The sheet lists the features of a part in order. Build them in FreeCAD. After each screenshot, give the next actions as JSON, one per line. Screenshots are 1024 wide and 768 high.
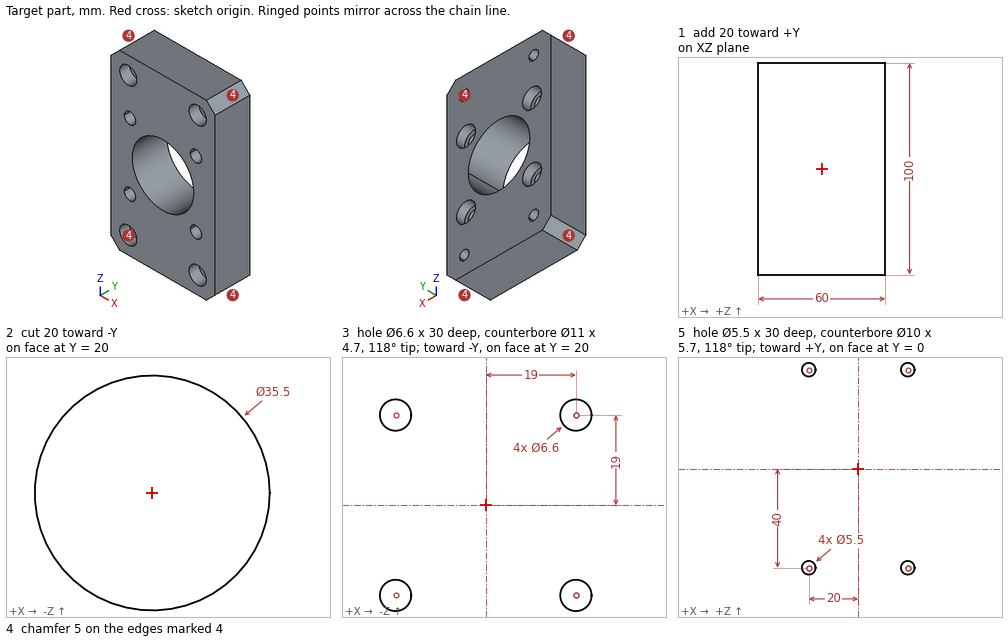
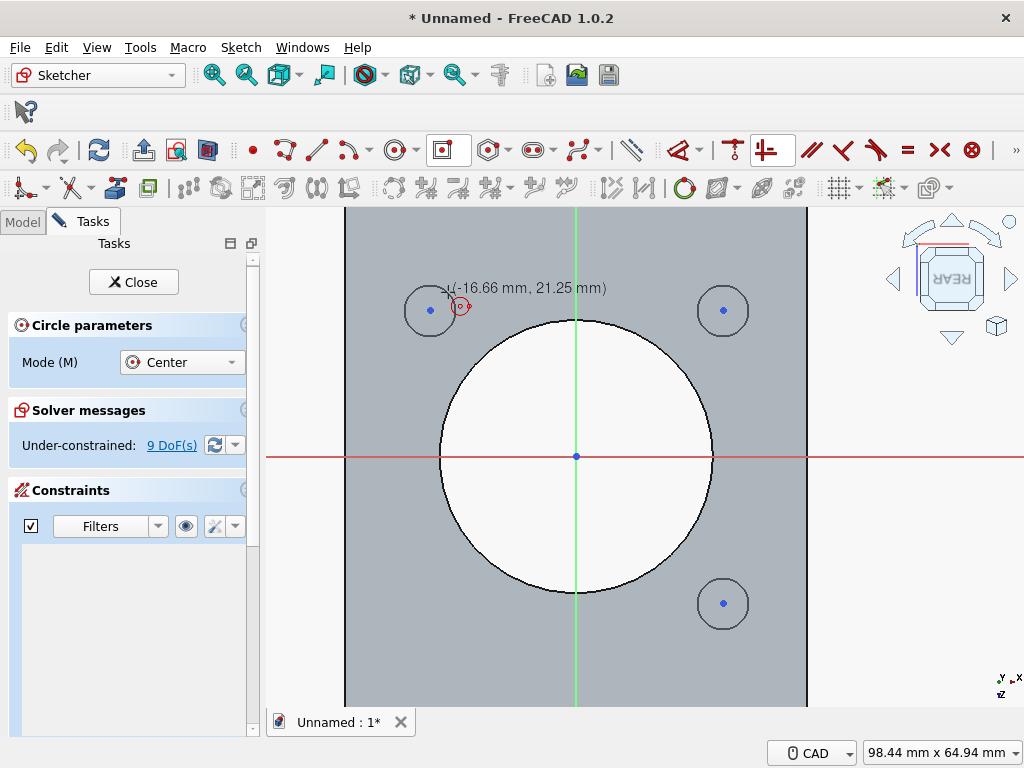
{"action": "left_click", "coordinate": [430, 603]}
{"action": "left_click", "coordinate": [448, 585]}
{"action": "key", "text": "Escape"}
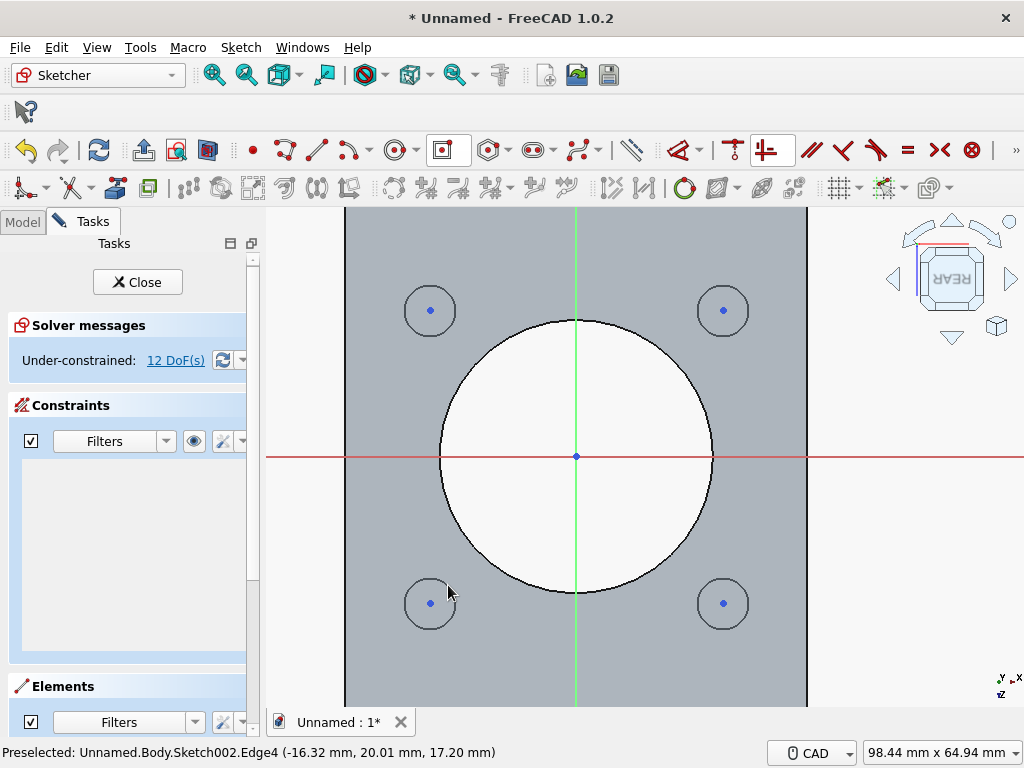
{"action": "left_click", "coordinate": [741, 293]}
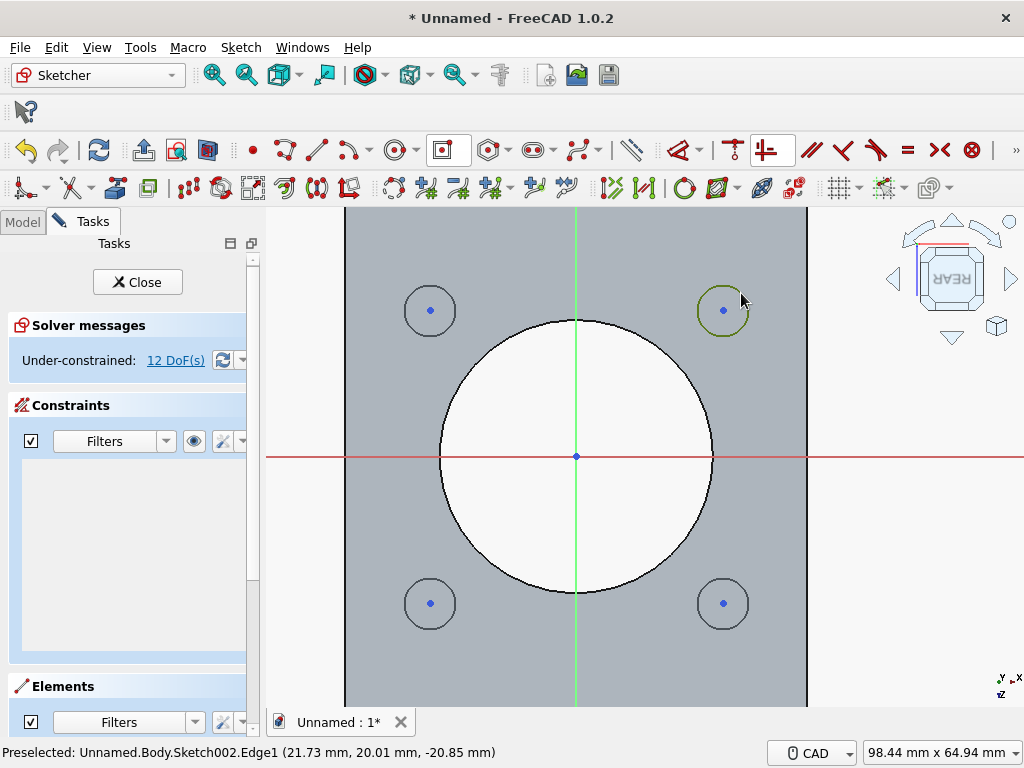
{"action": "left_click", "coordinate": [741, 586]}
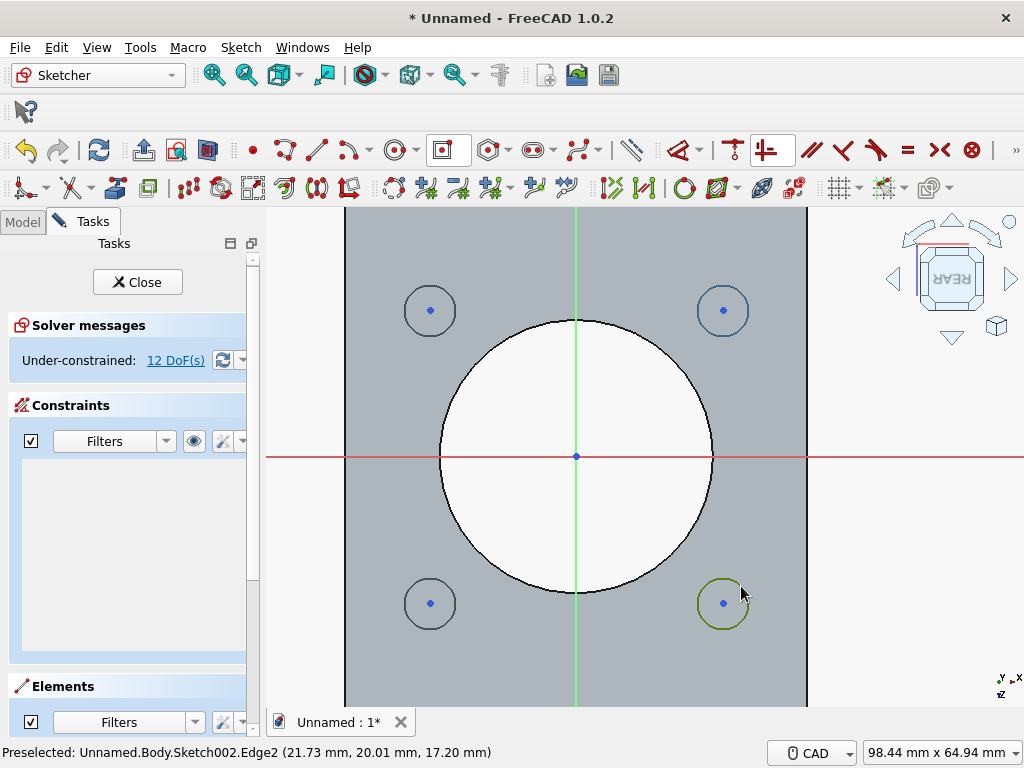
{"action": "left_click", "coordinate": [448, 293]}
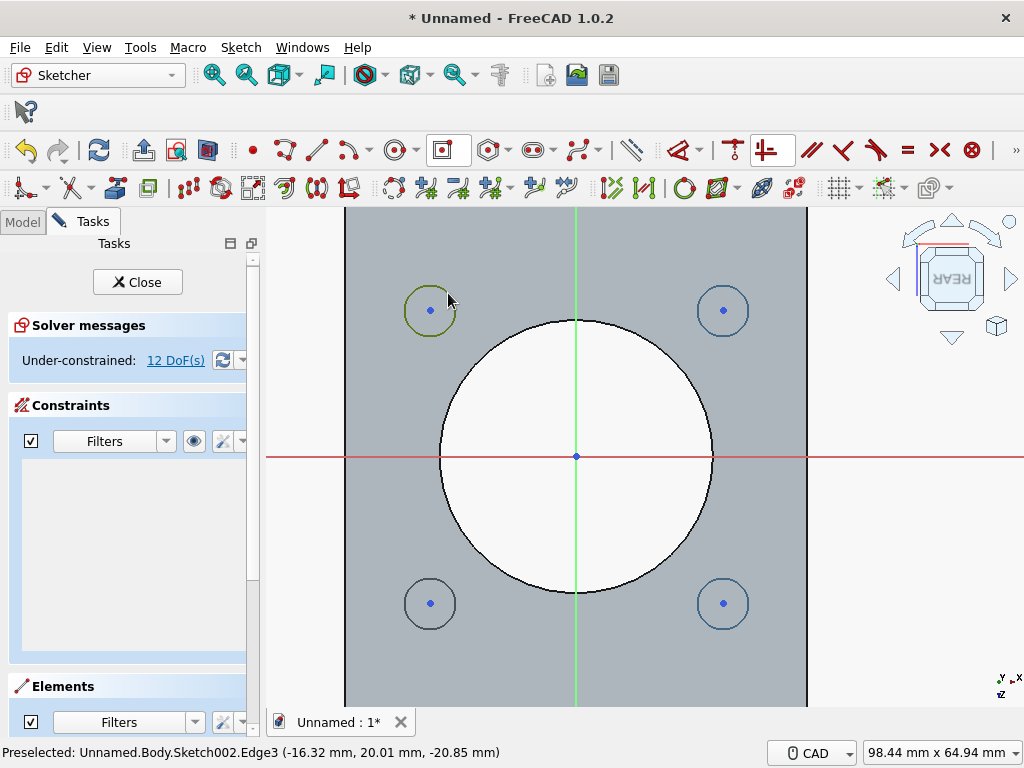
{"action": "left_click", "coordinate": [448, 586]}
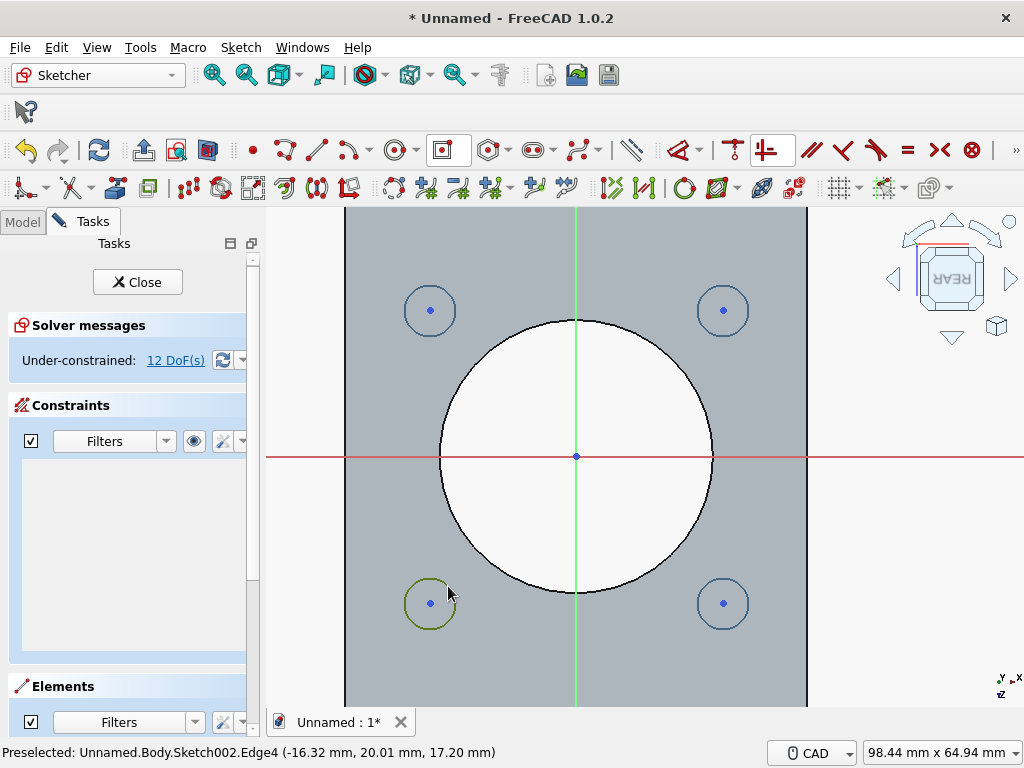
{"action": "left_click", "coordinate": [908, 150]}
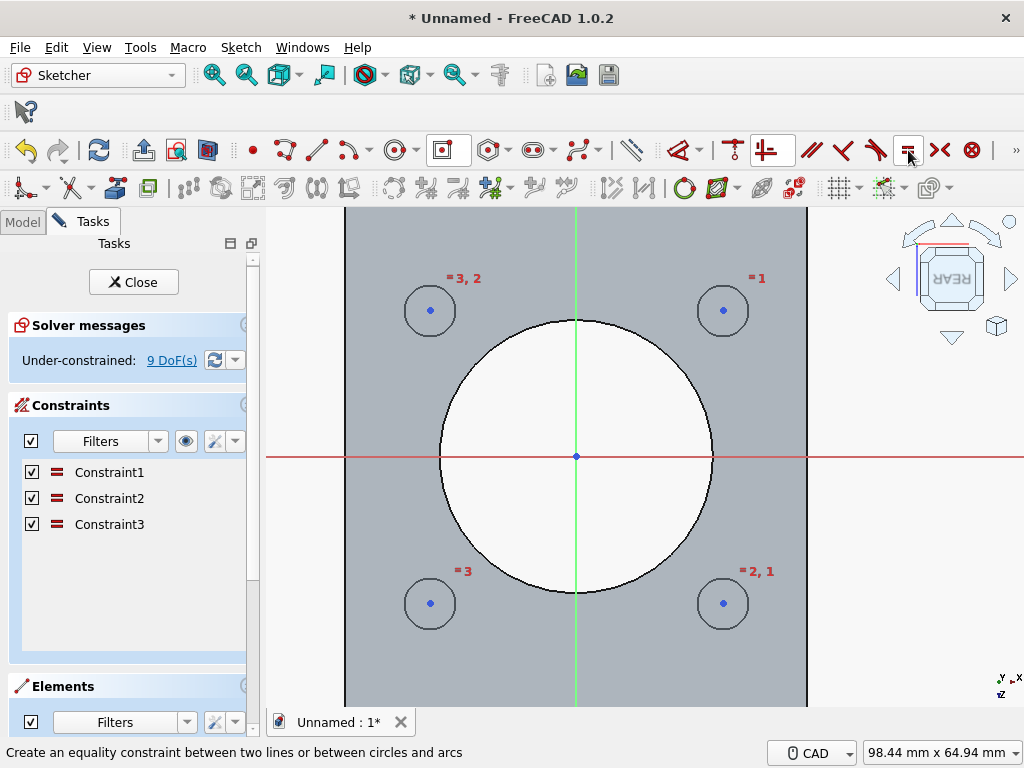
{"action": "left_click", "coordinate": [723, 311]}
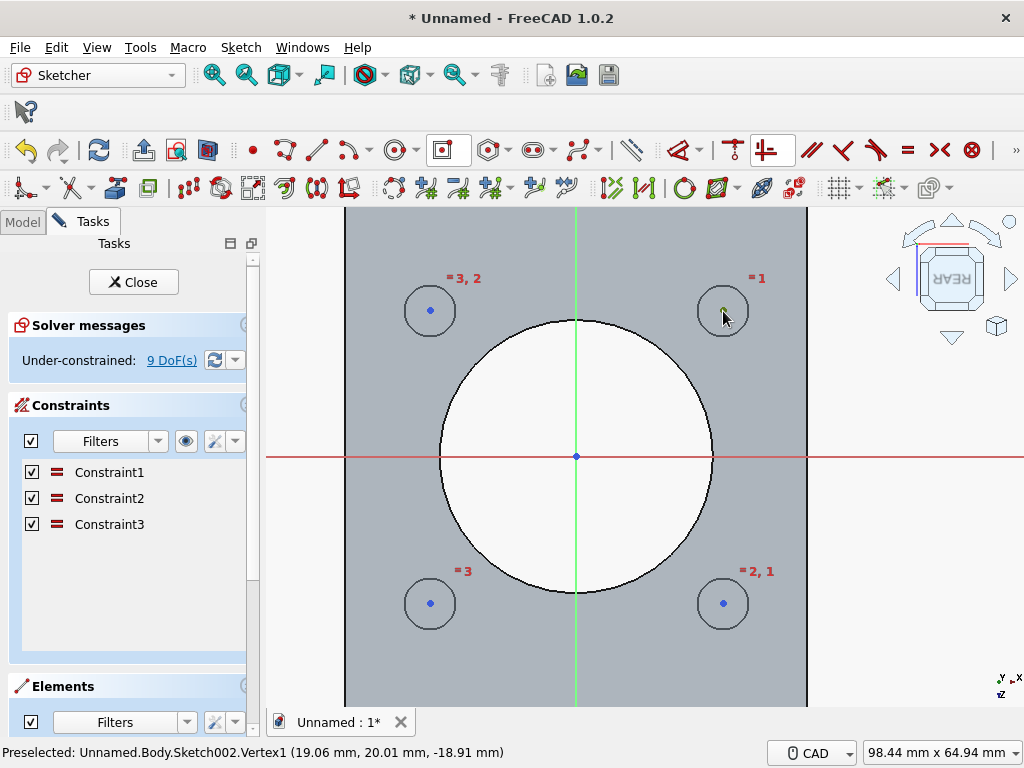
{"action": "left_click", "coordinate": [723, 604]}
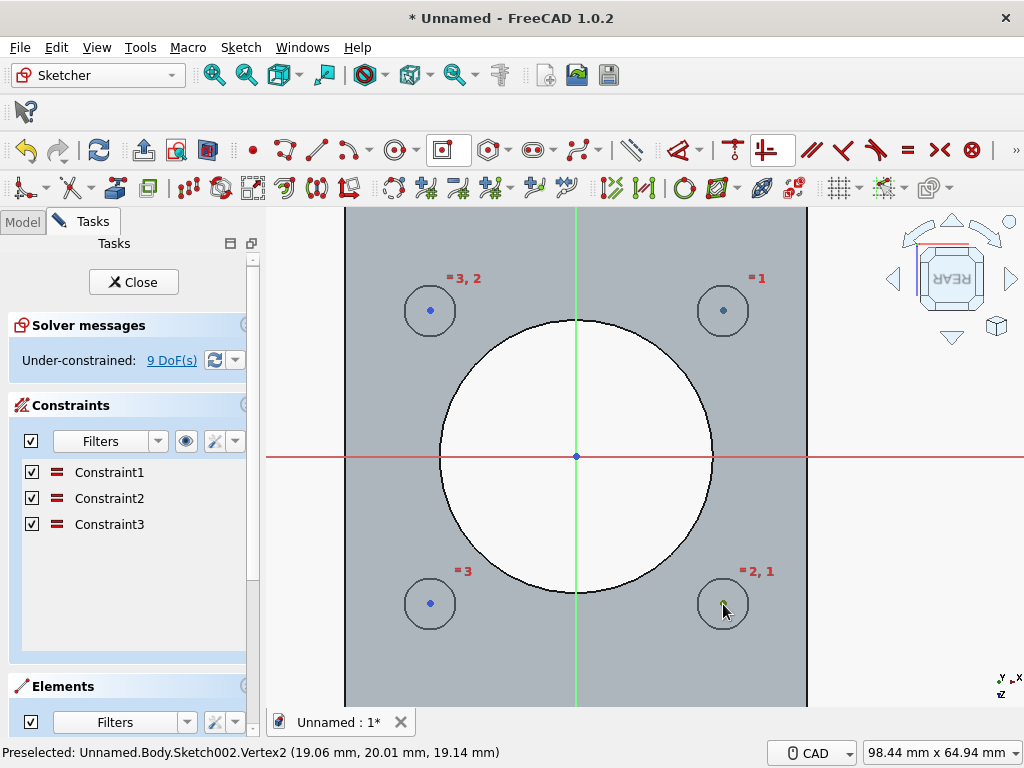
{"action": "left_click", "coordinate": [334, 457]}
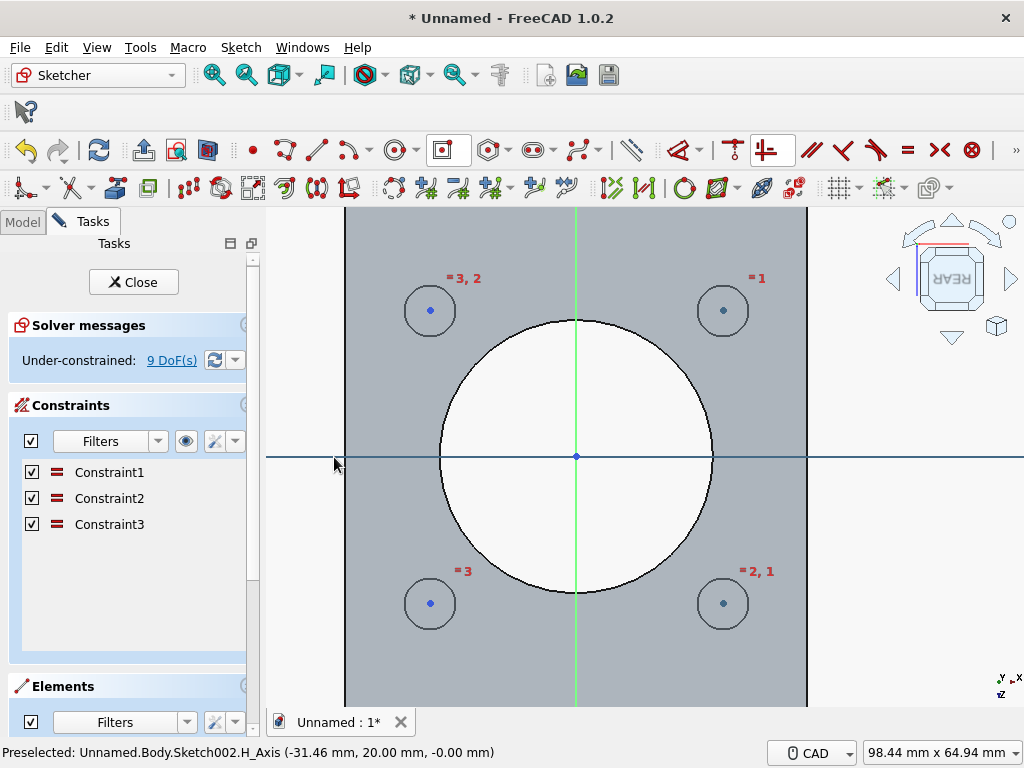
{"action": "left_click", "coordinate": [940, 150]}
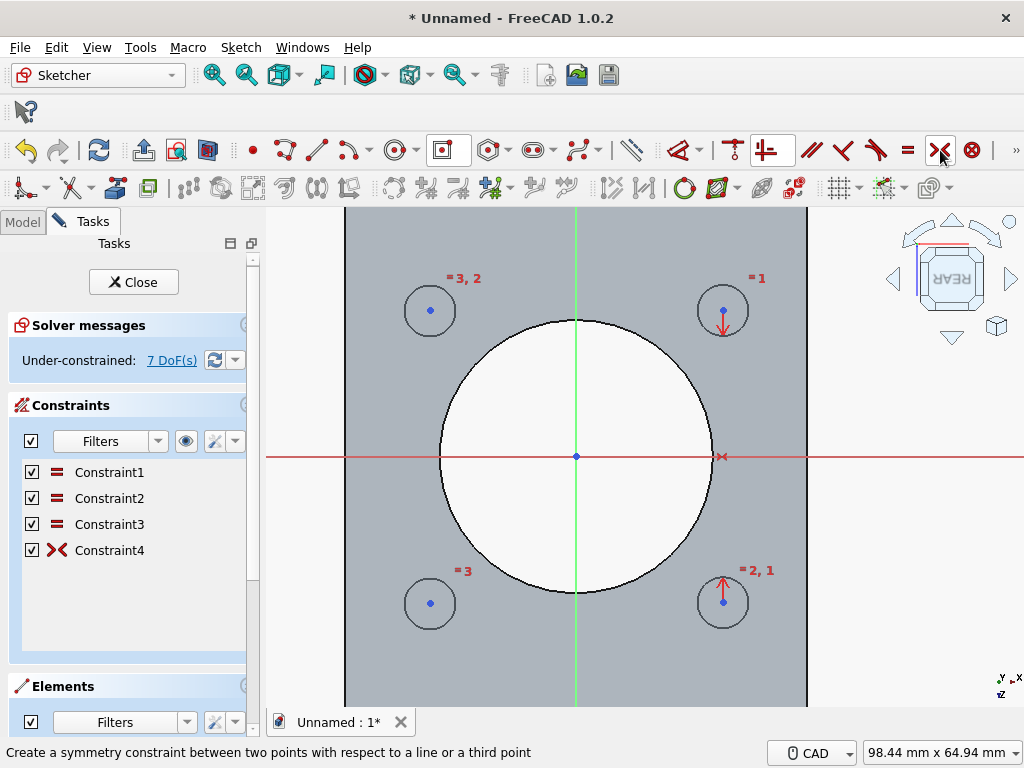
{"action": "left_click", "coordinate": [723, 310]}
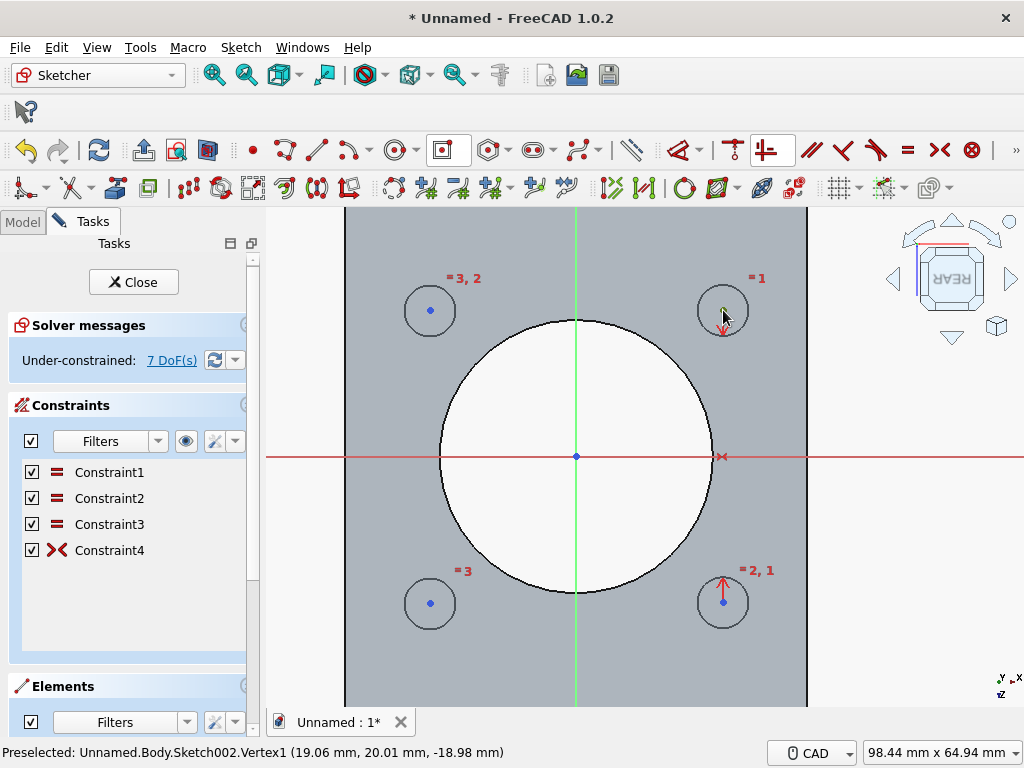
{"action": "left_click", "coordinate": [430, 311]}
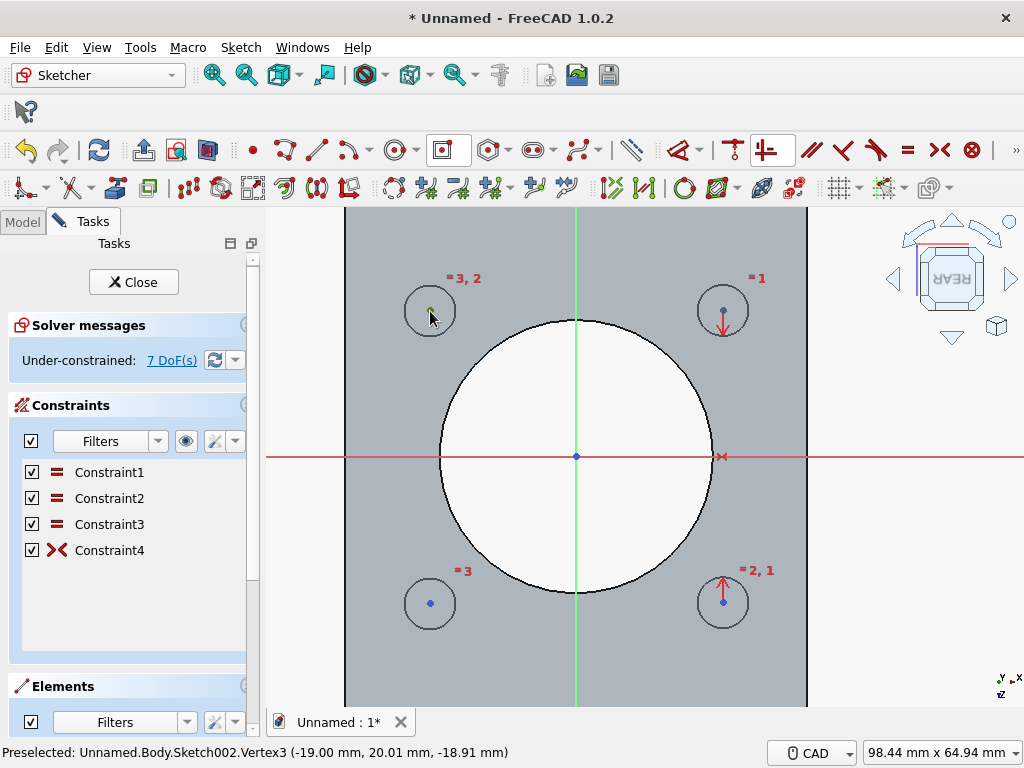
{"action": "left_click", "coordinate": [576, 647]}